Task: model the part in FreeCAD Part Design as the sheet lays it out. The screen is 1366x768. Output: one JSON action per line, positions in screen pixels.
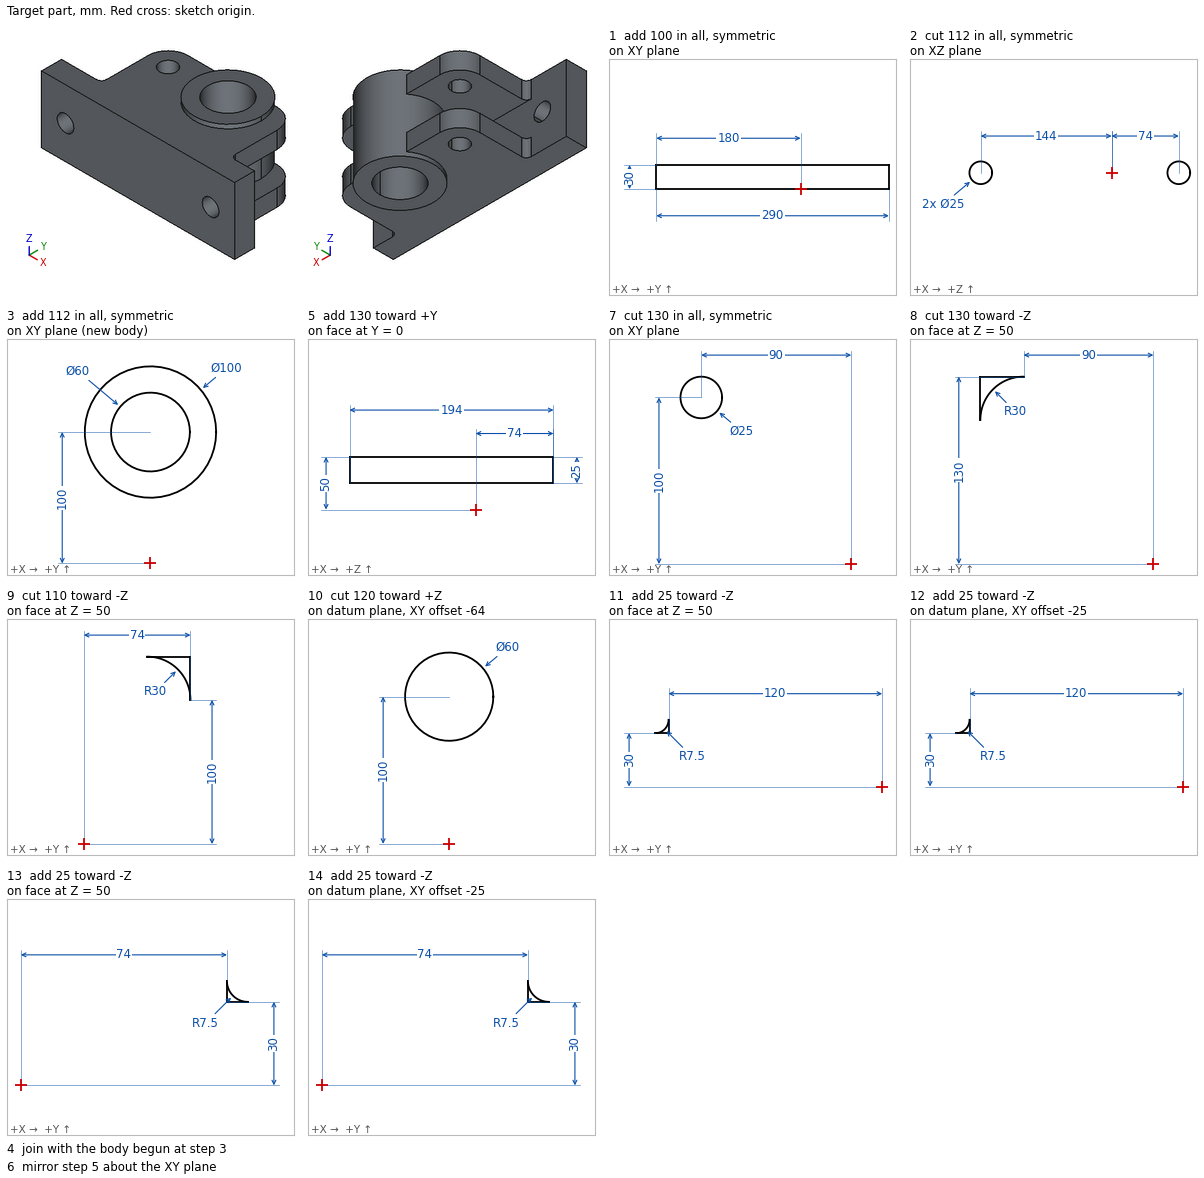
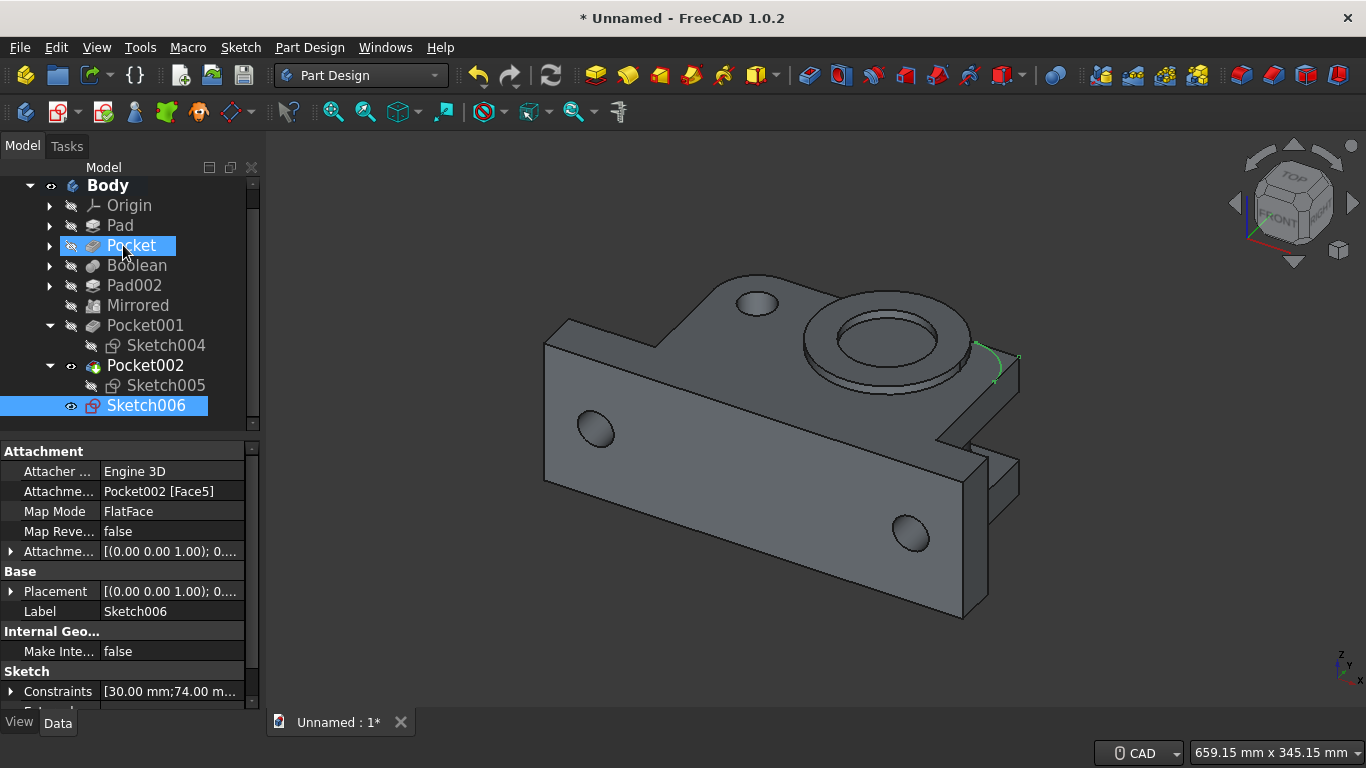
{"action": "left_click", "coordinate": [810, 76]}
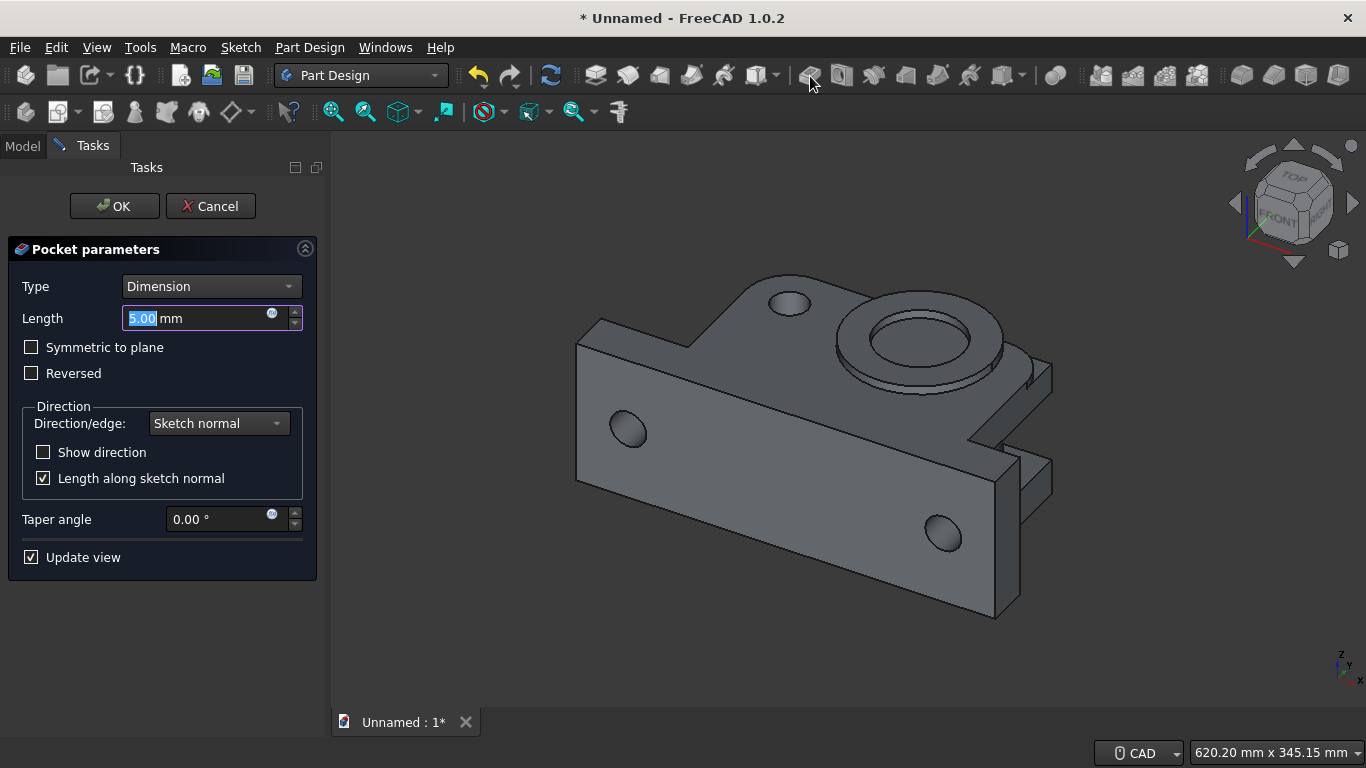
{"action": "type", "text": "110"}
{"action": "key", "text": "Tab"}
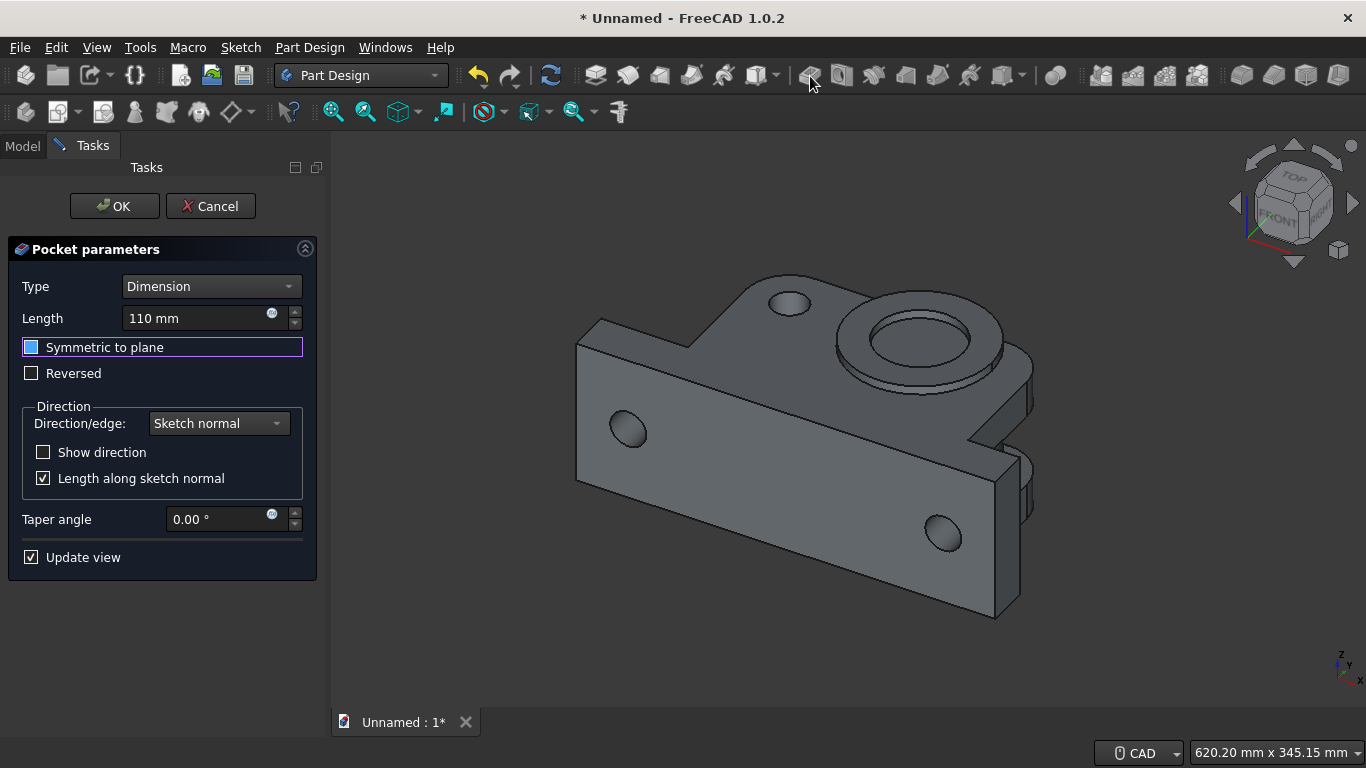
{"action": "left_click", "coordinate": [115, 206]}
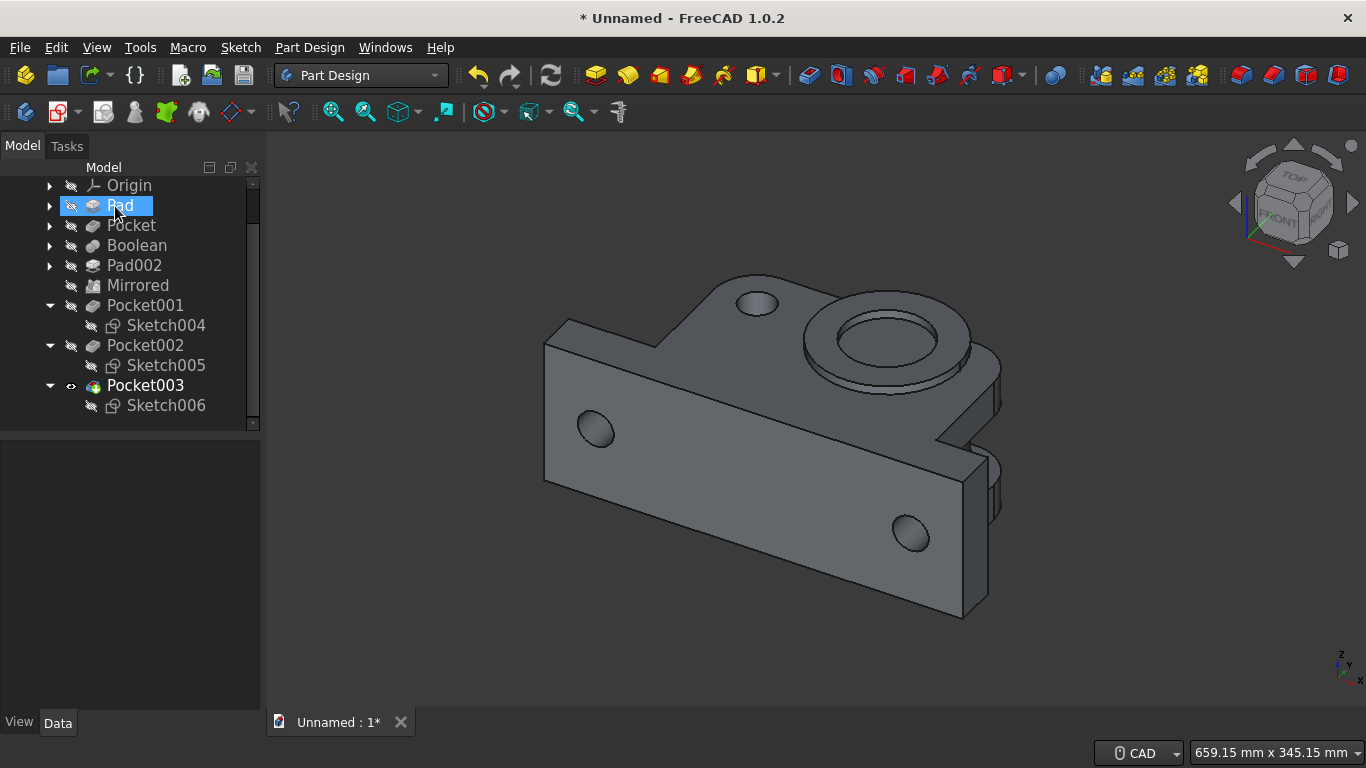
{"action": "left_click", "coordinate": [50, 186]}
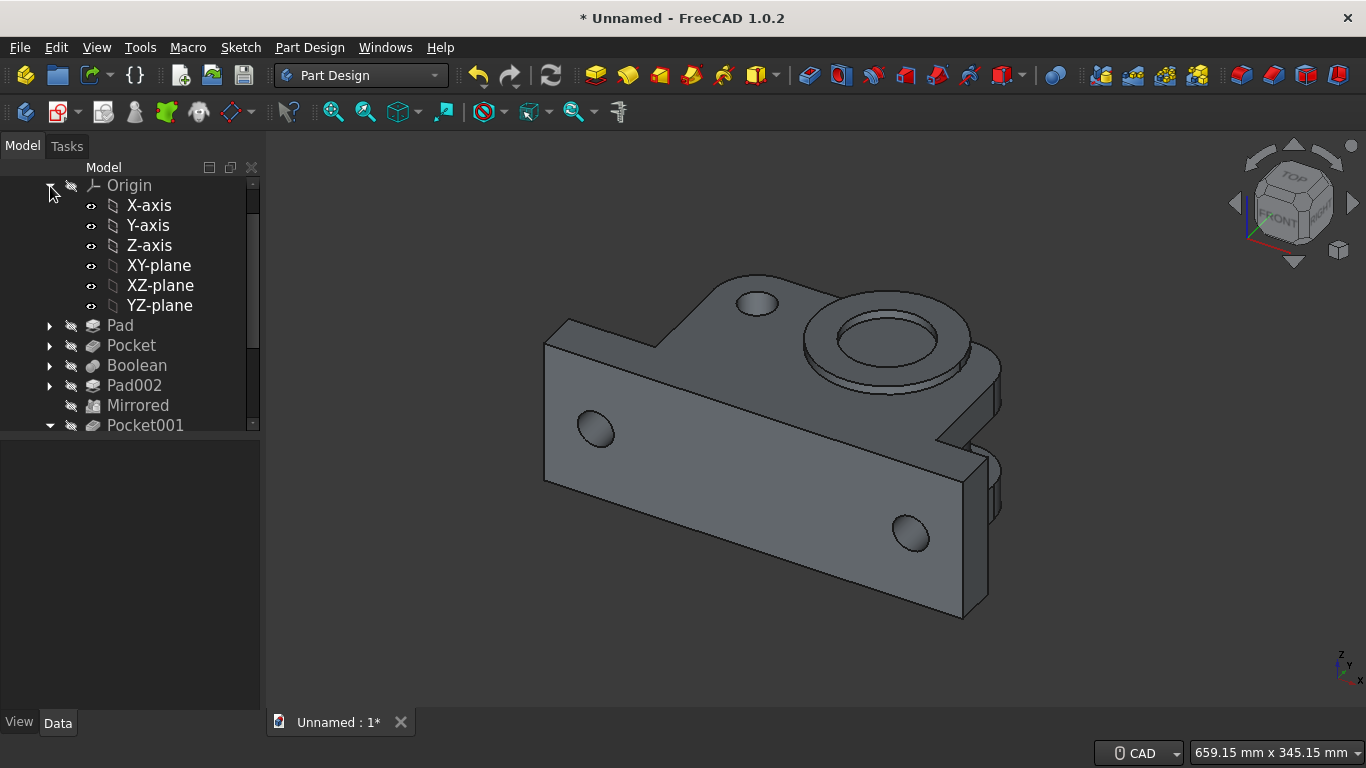
{"action": "left_click", "coordinate": [136, 266]}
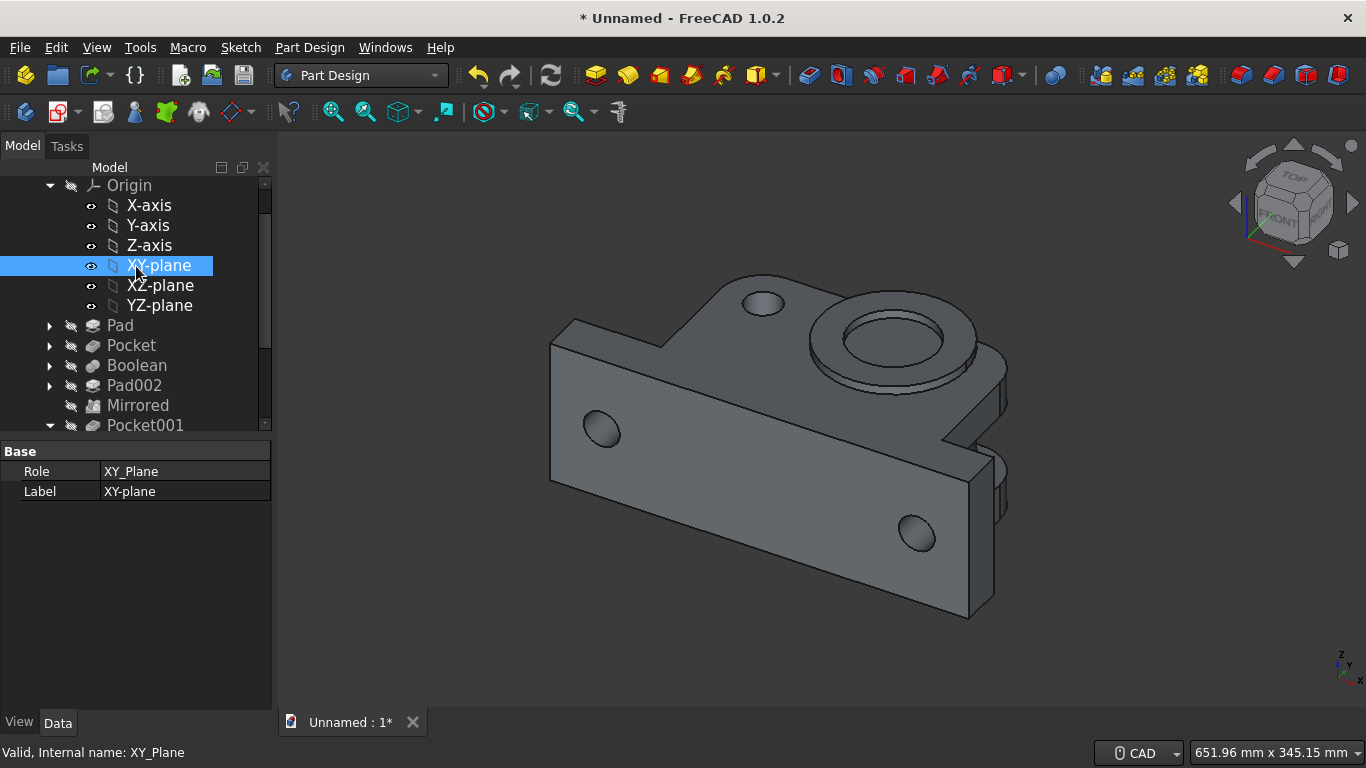
{"action": "left_click", "coordinate": [232, 112]}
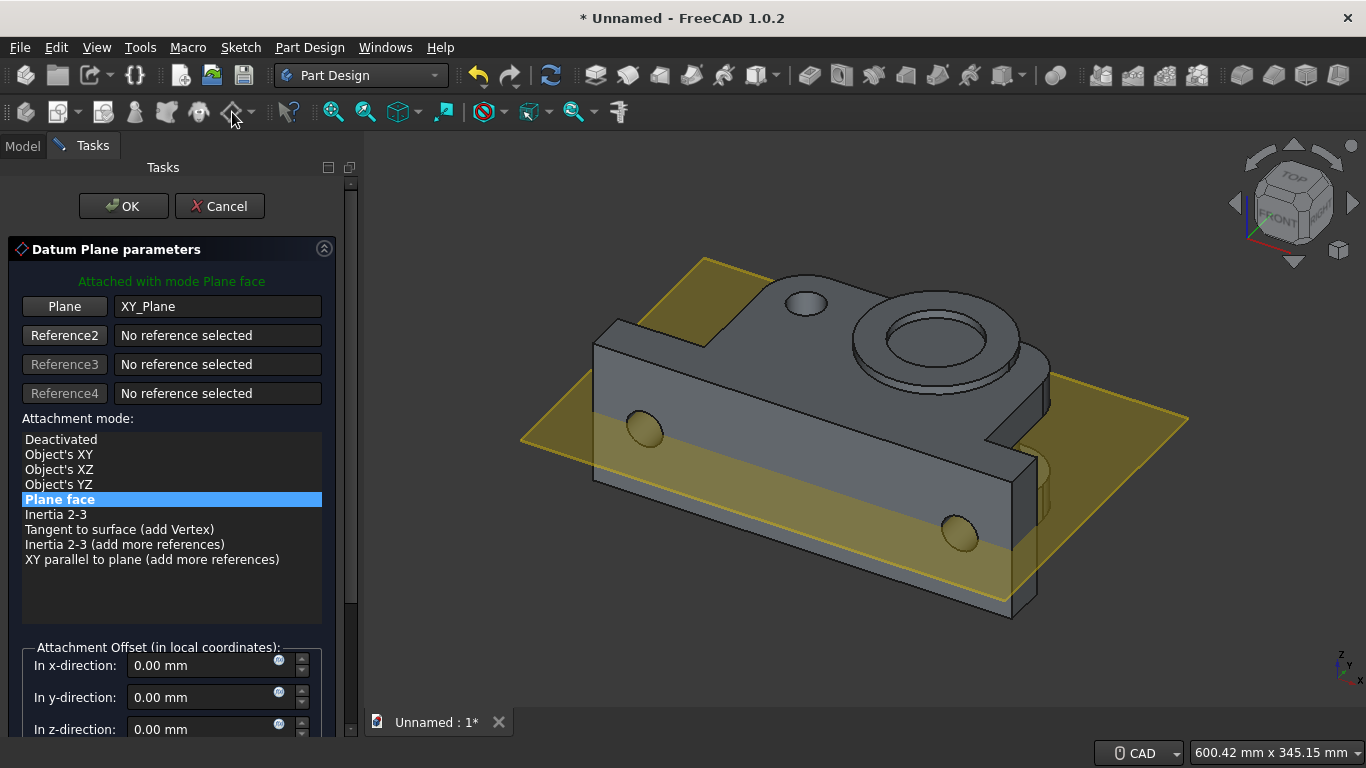
{"action": "scroll", "coordinate": [351, 456], "scroll_direction": "down", "scroll_amount": 2}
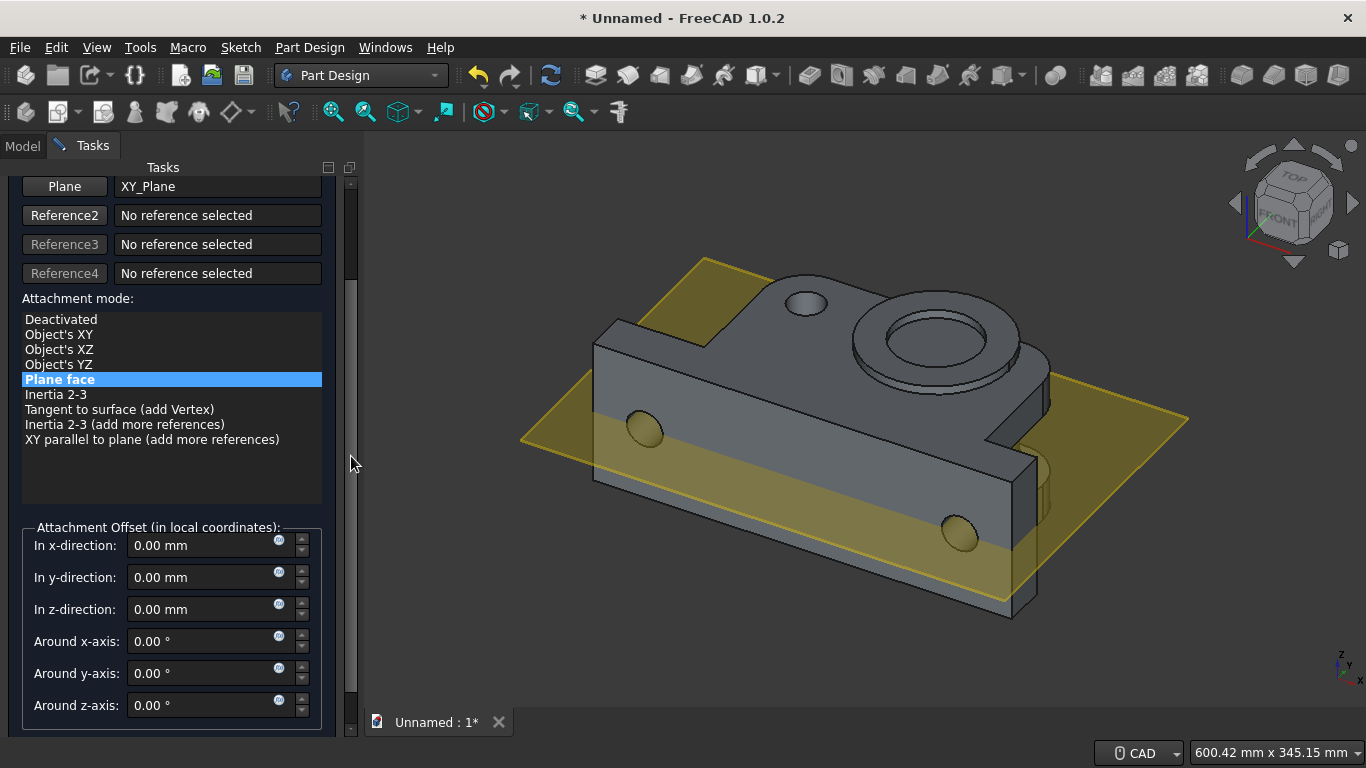
{"action": "triple_click", "coordinate": [210, 609]}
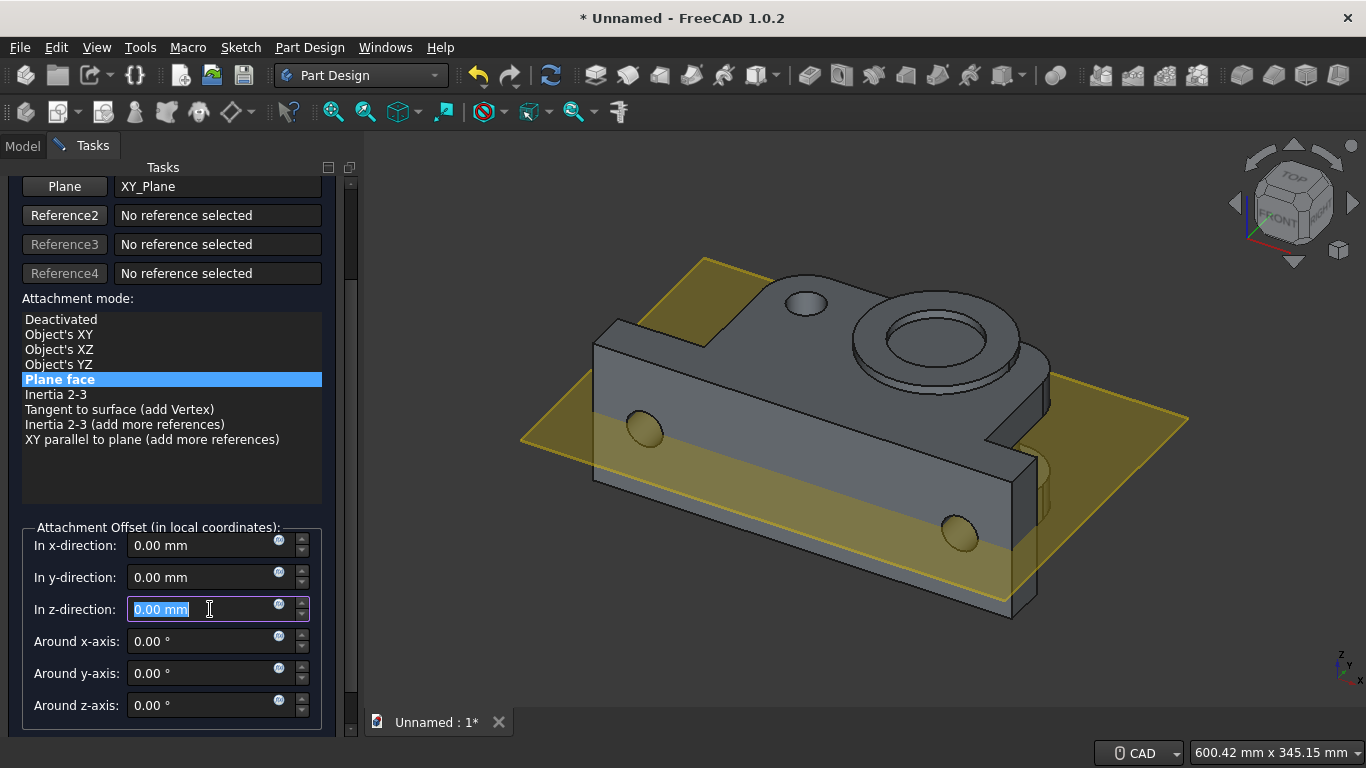
{"action": "type", "text": "-64"}
{"action": "key", "text": "Tab"}